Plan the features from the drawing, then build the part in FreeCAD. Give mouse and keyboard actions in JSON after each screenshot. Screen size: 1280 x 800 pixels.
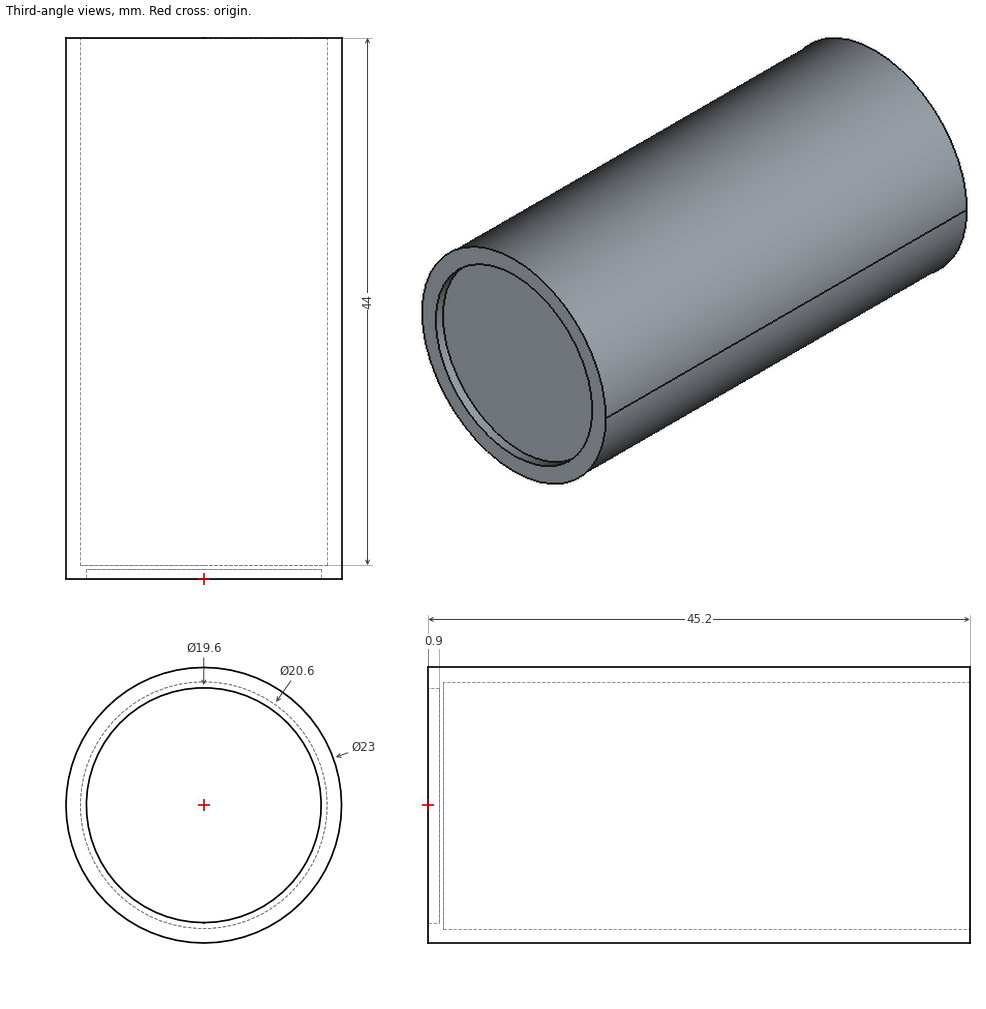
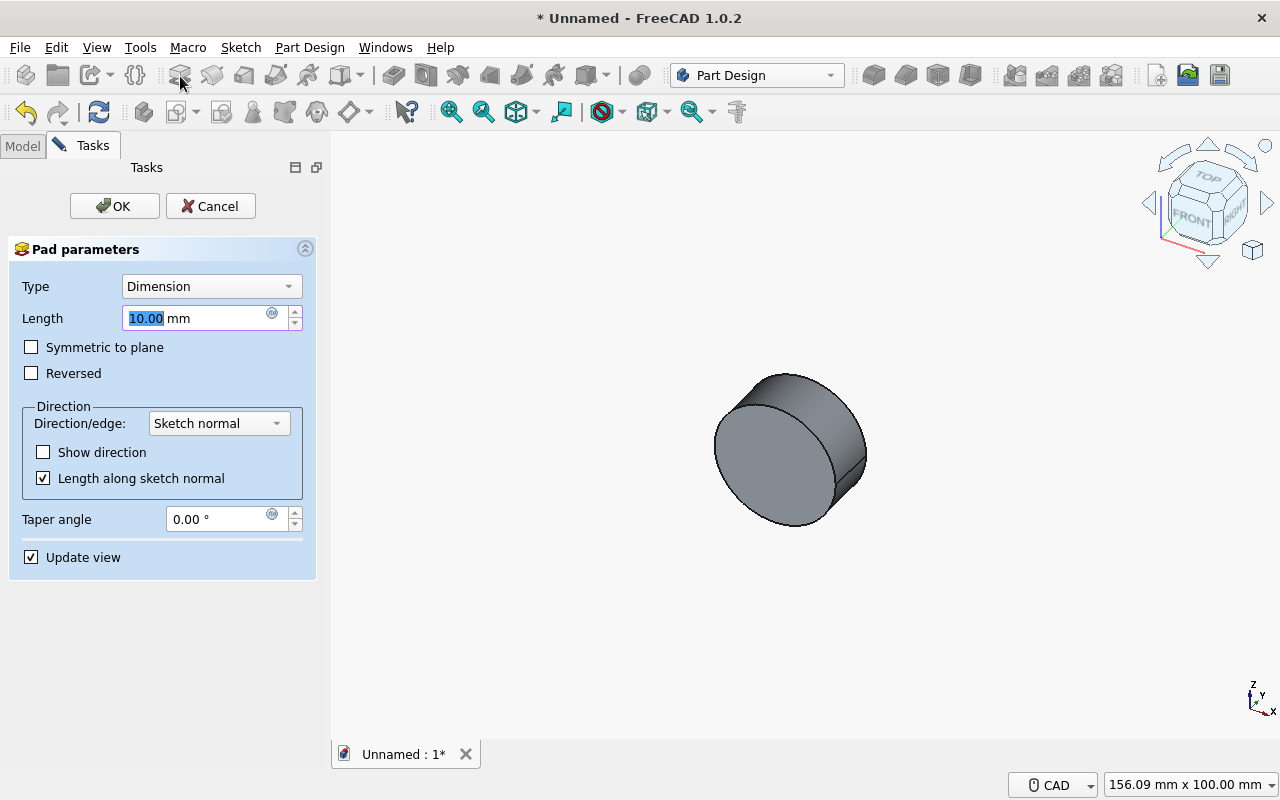
{"action": "type", "text": "45.2"}
{"action": "key", "text": "Tab"}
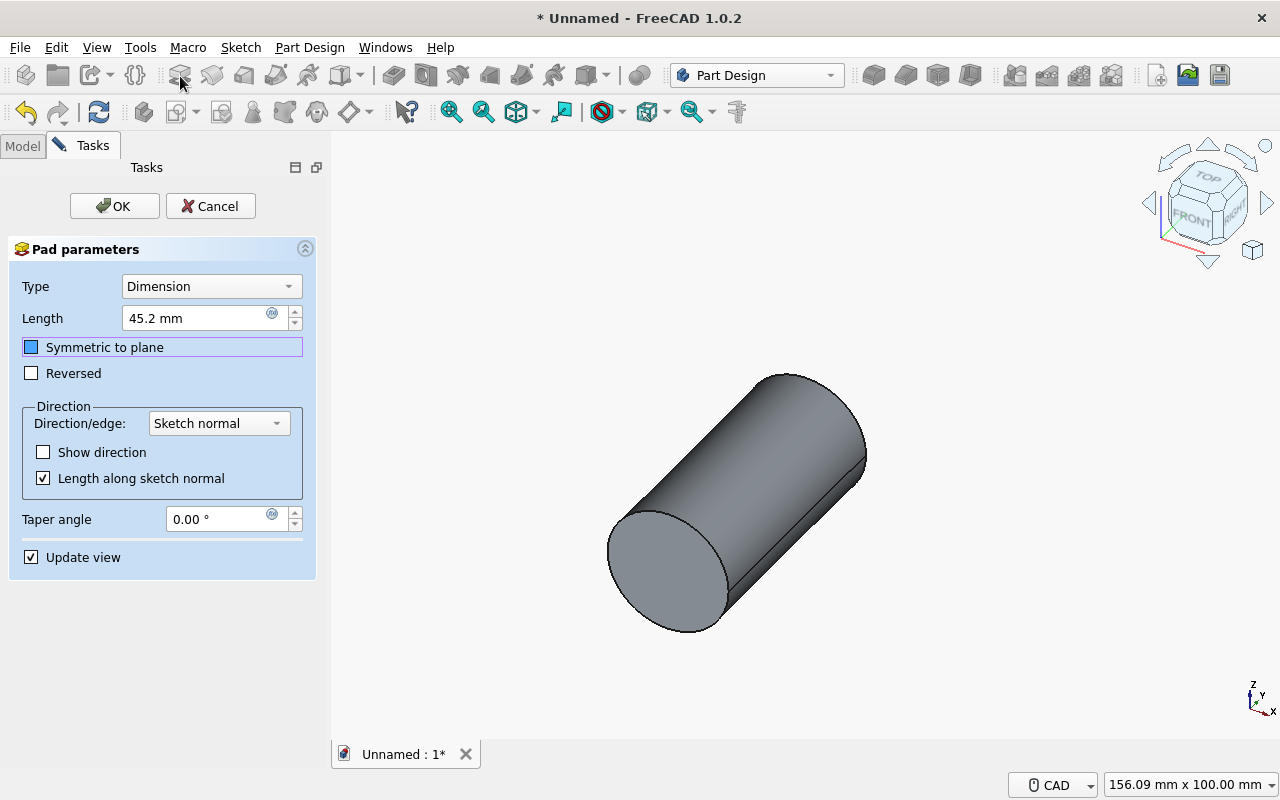
{"action": "left_click", "coordinate": [30, 373]}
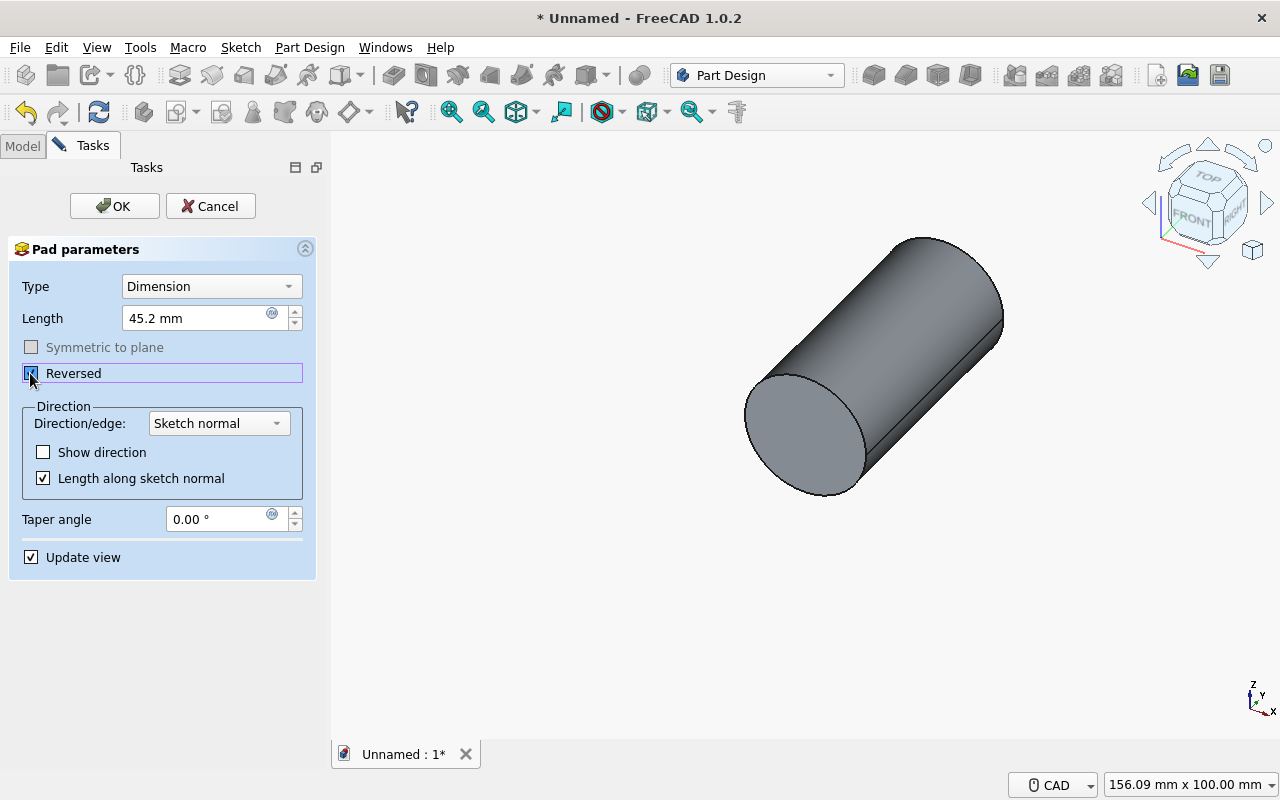
{"action": "left_click", "coordinate": [115, 206]}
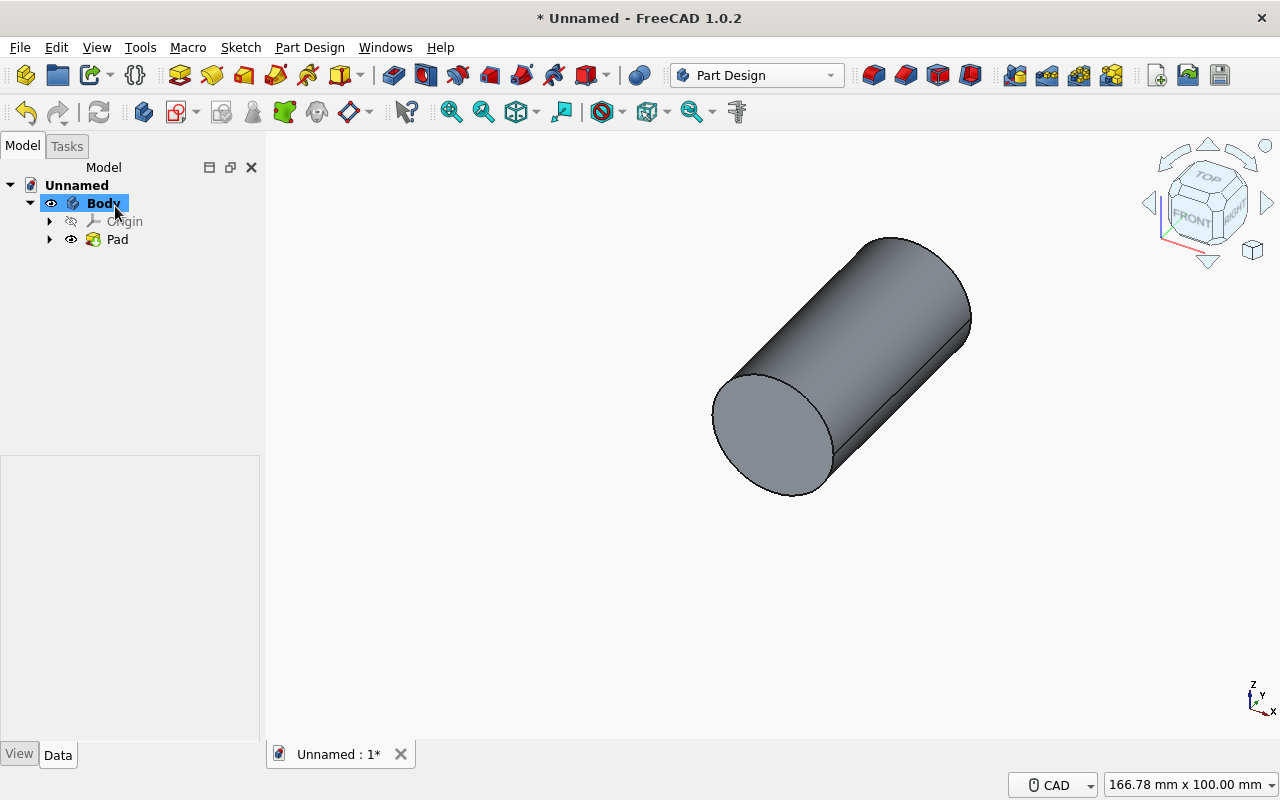
{"action": "key", "text": "4"}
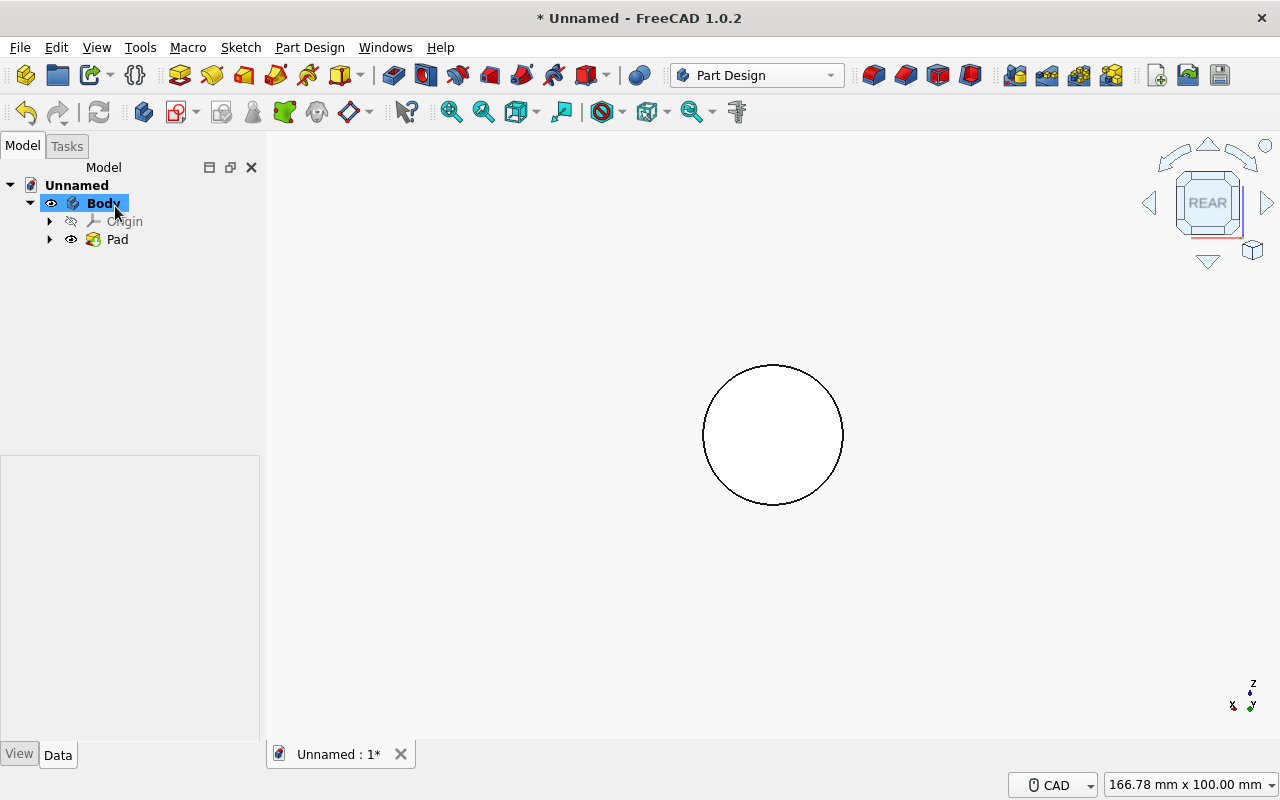
{"action": "left_click", "coordinate": [452, 112]}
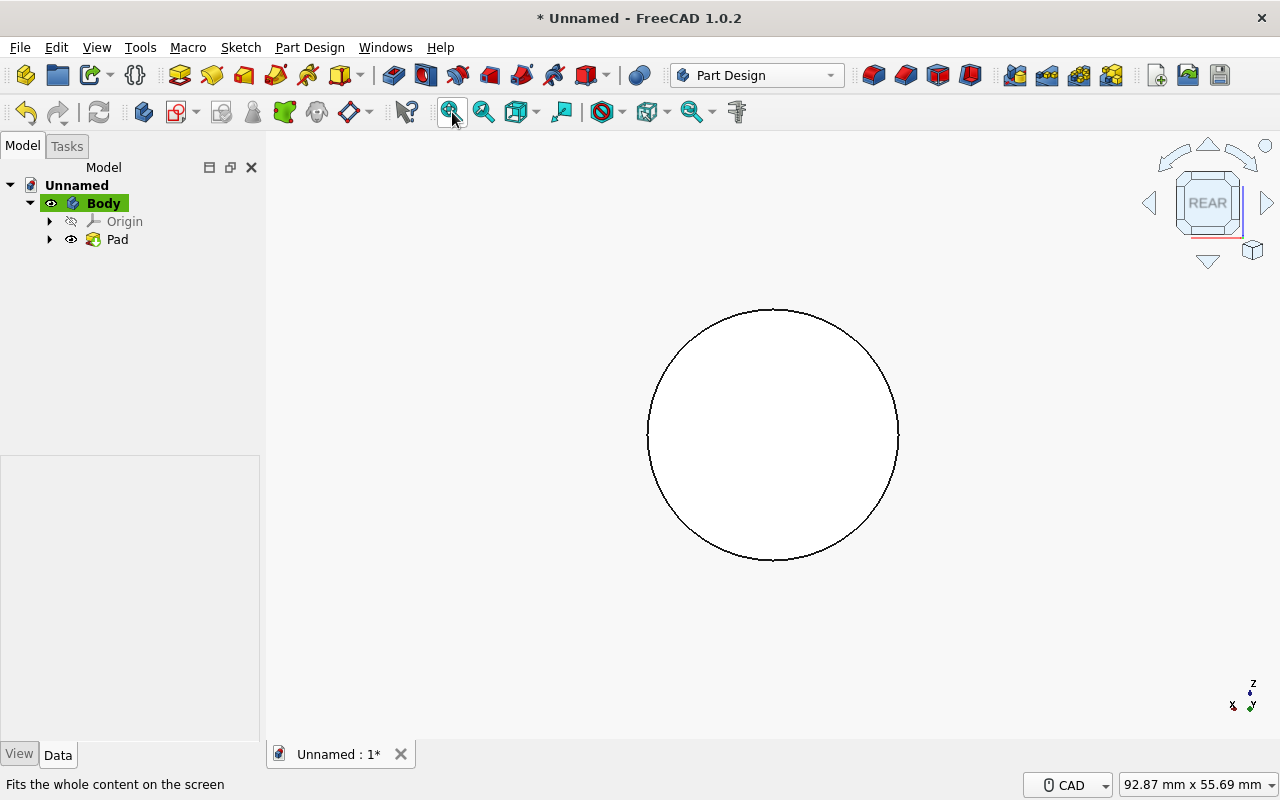
{"action": "left_click", "coordinate": [773, 434]}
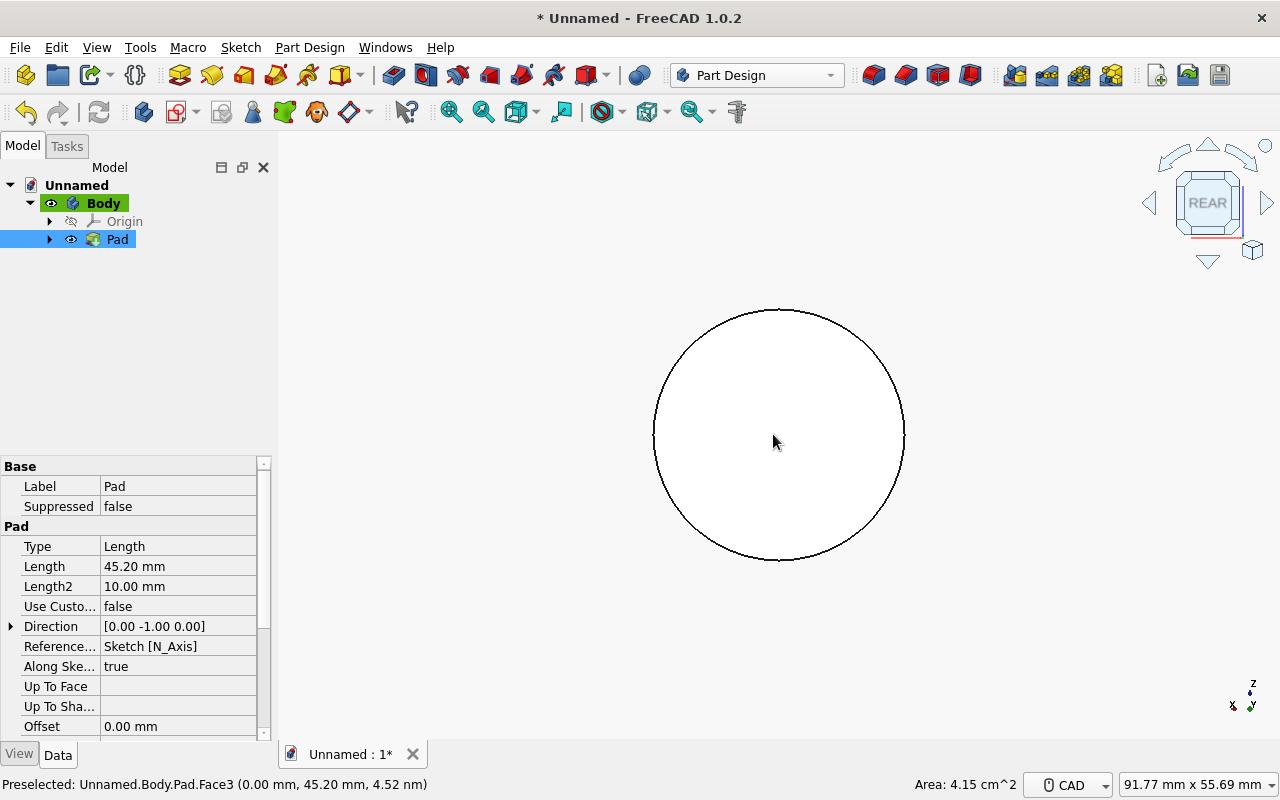
{"action": "left_click", "coordinate": [176, 112]}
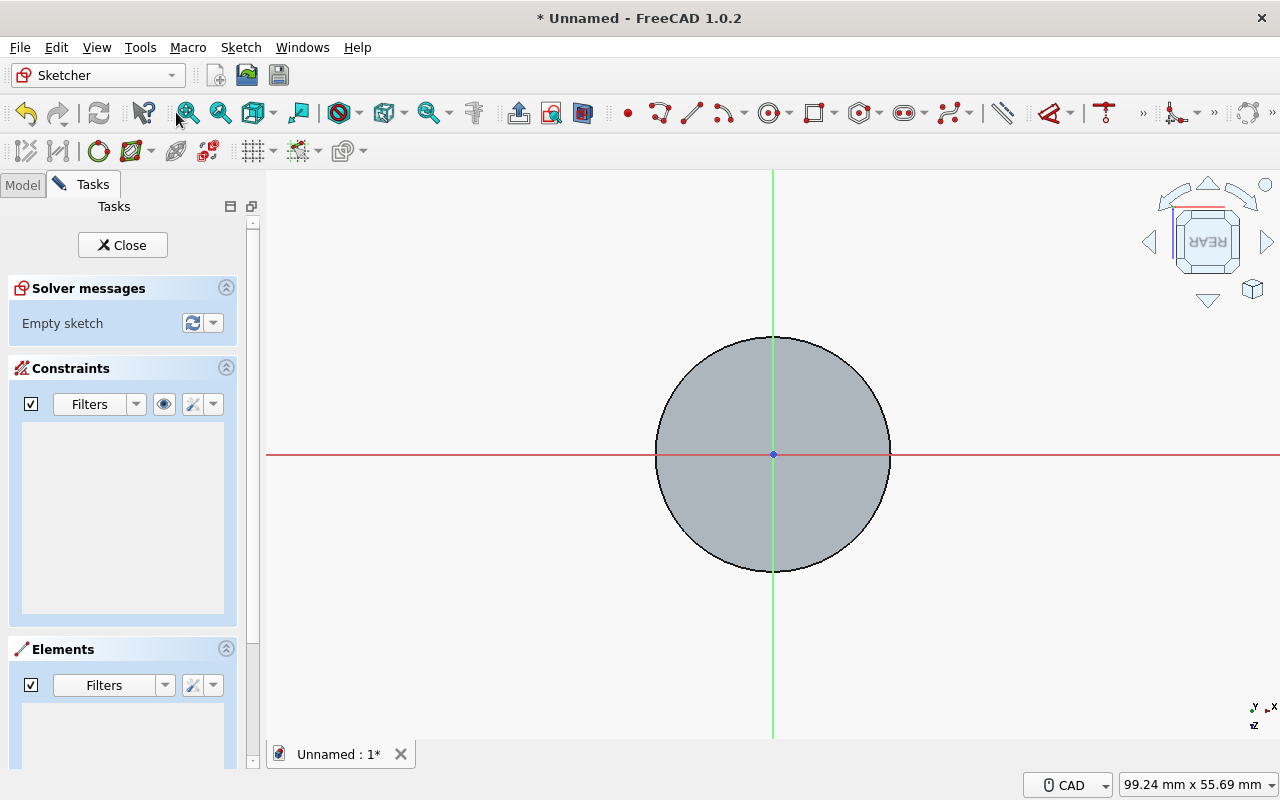
{"action": "scroll", "coordinate": [856, 454], "scroll_direction": "up", "scroll_amount": 3}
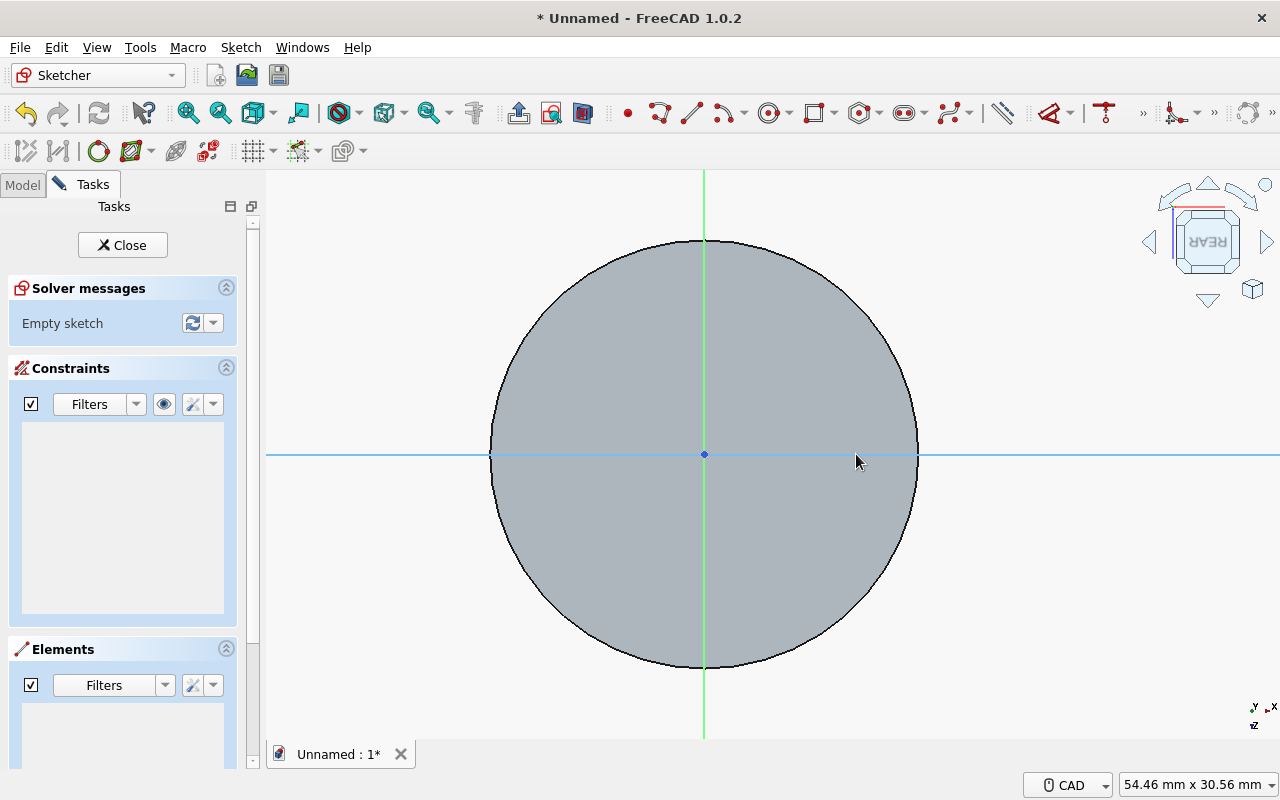
{"action": "left_click", "coordinate": [770, 114]}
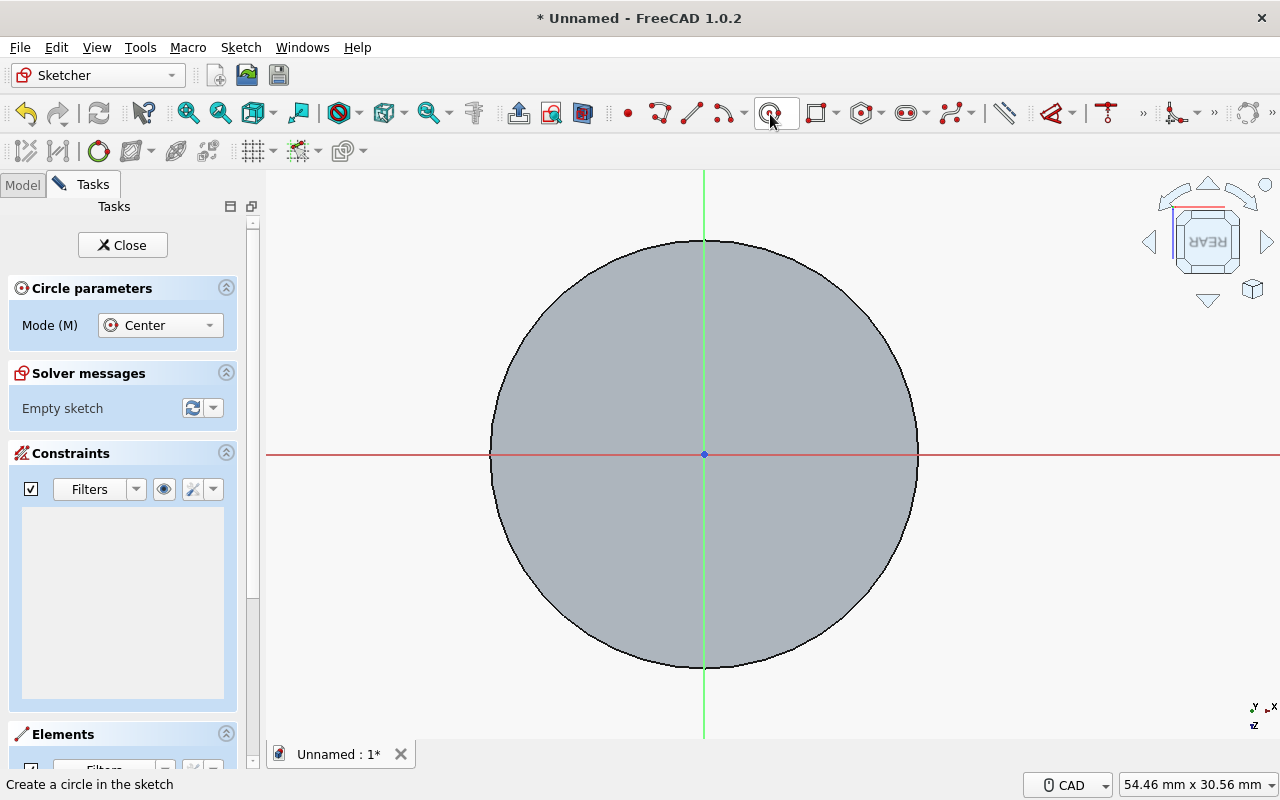
{"action": "left_click", "coordinate": [704, 454]}
{"action": "mouse_move", "coordinate": [840, 319]}